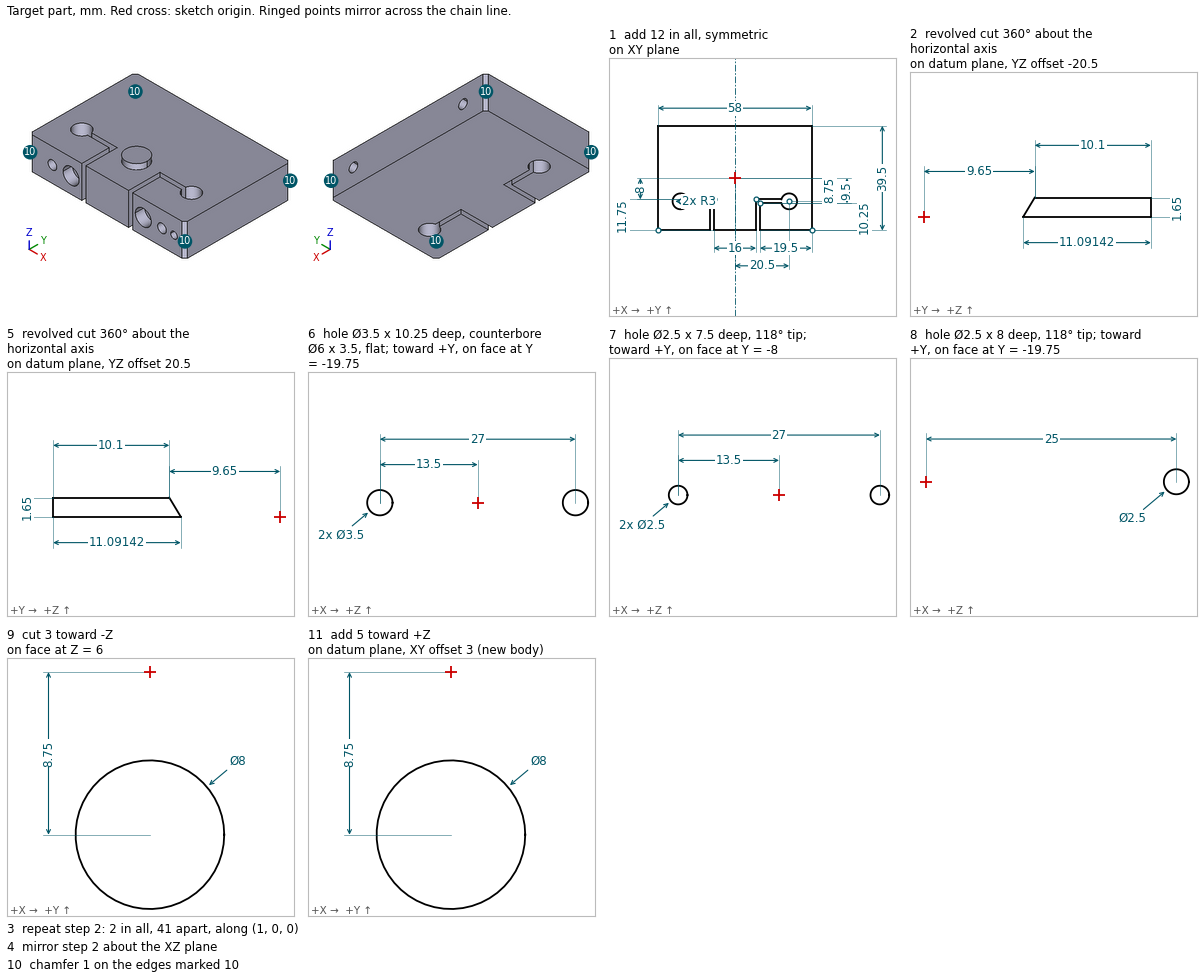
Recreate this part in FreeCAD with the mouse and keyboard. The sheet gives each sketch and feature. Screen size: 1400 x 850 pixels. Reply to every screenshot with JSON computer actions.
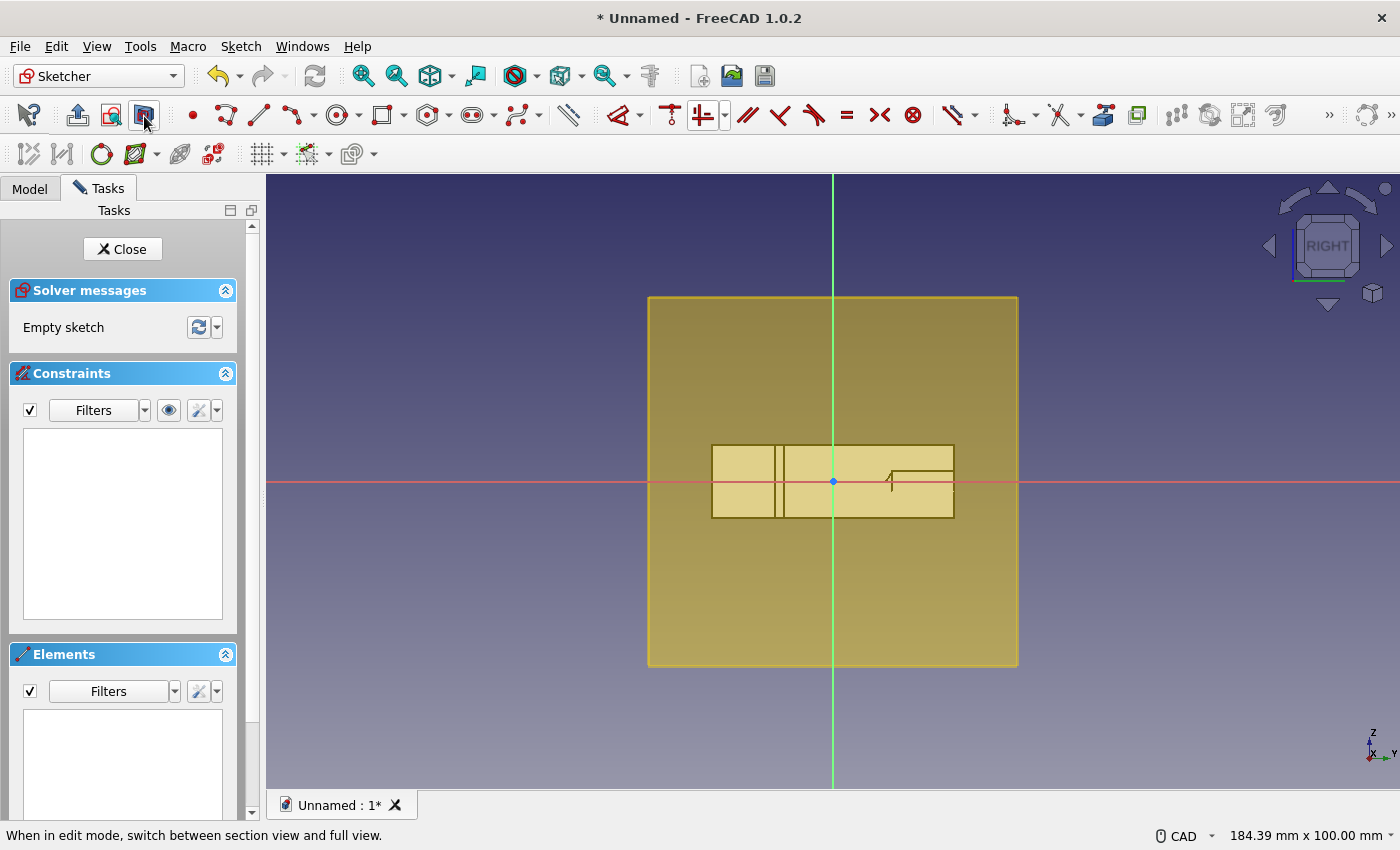
{"action": "scroll", "coordinate": [774, 475], "scroll_direction": "up", "scroll_amount": 8}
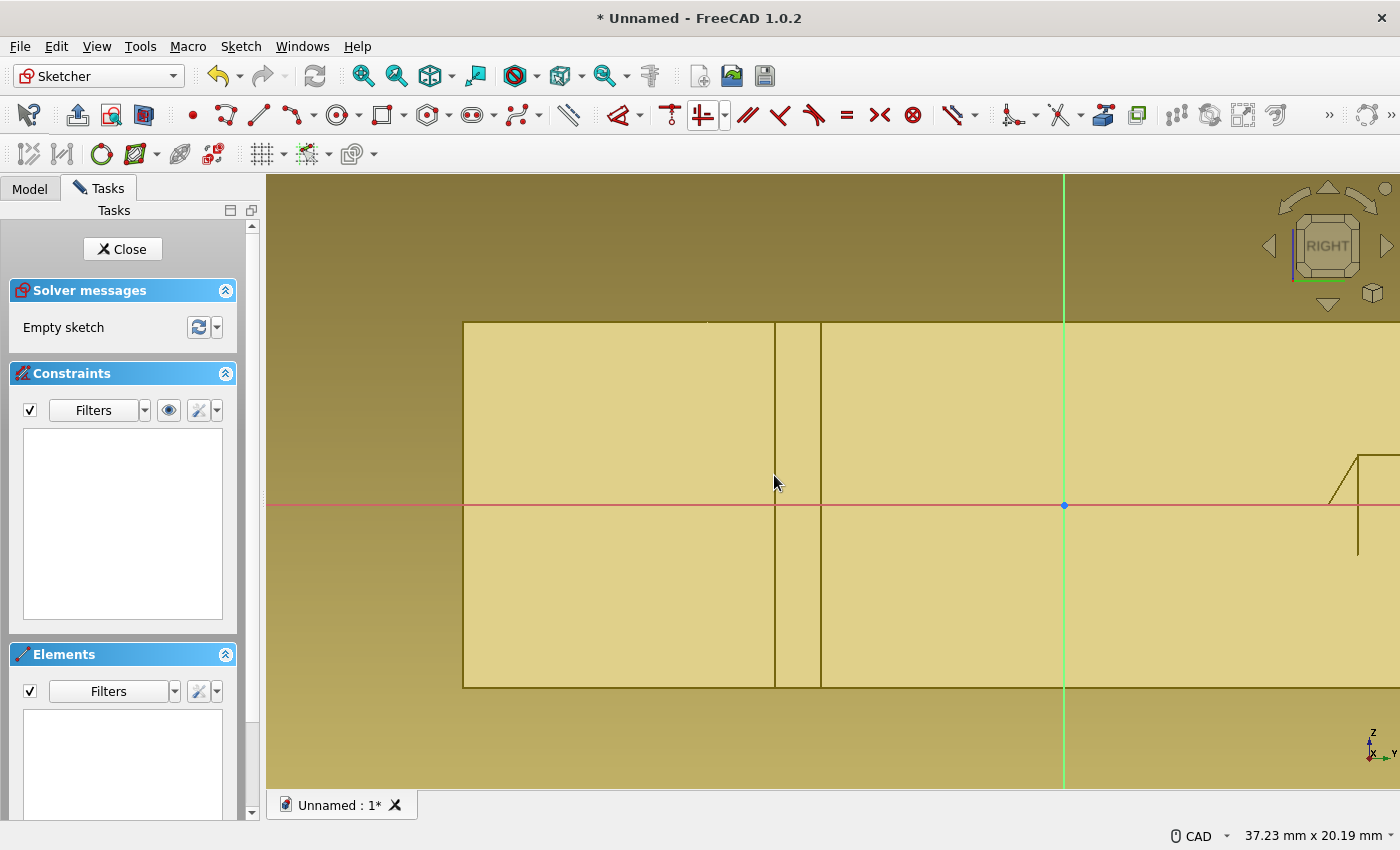
{"action": "left_click", "coordinate": [226, 116]}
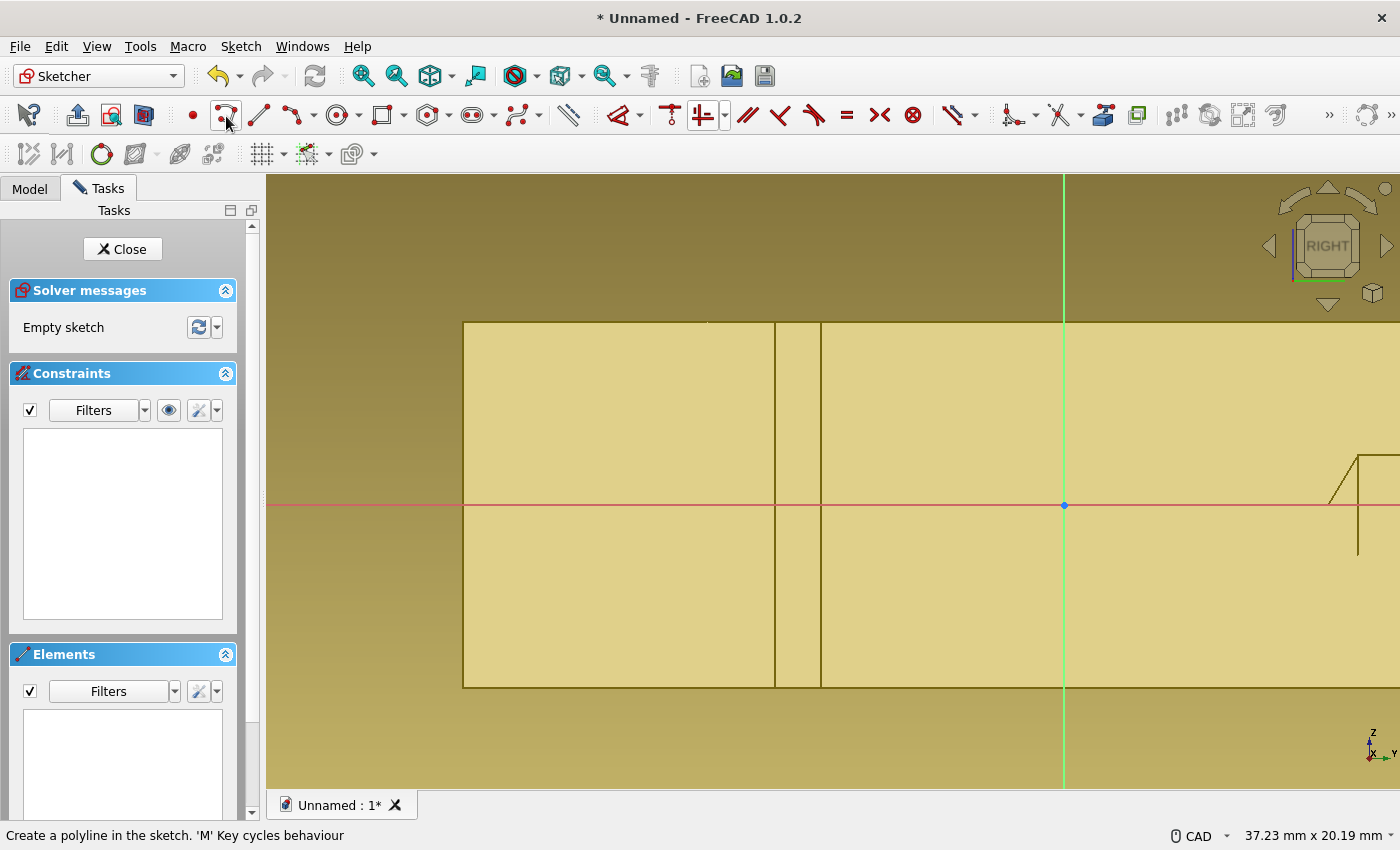
{"action": "left_click", "coordinate": [801, 505]}
{"action": "left_click", "coordinate": [771, 455]}
{"action": "left_click", "coordinate": [463, 455]}
{"action": "left_click", "coordinate": [463, 496]}
{"action": "left_click", "coordinate": [801, 505]}
{"action": "key", "text": "Escape"}
{"action": "key", "text": "Escape"}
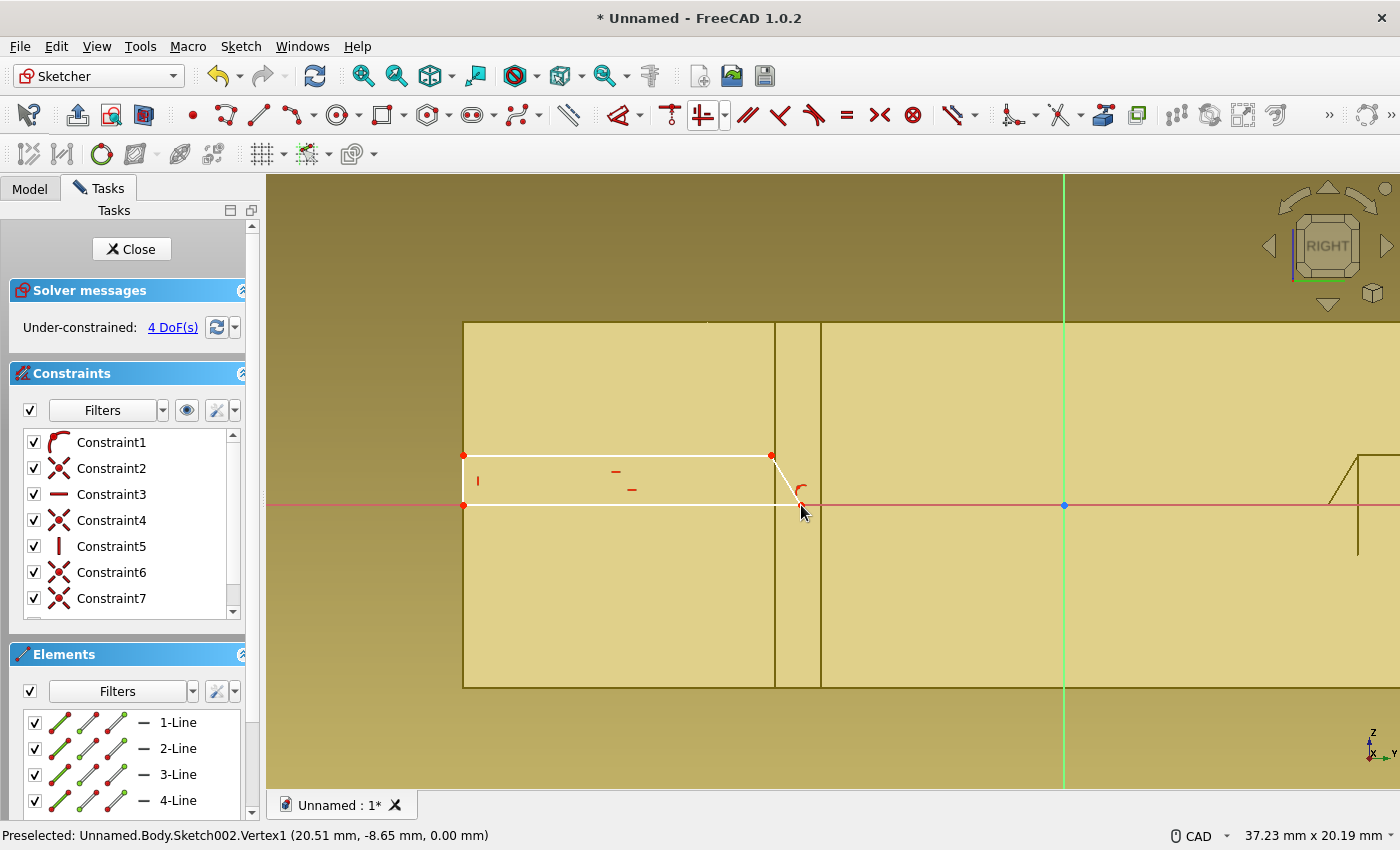
{"action": "left_click", "coordinate": [618, 116]}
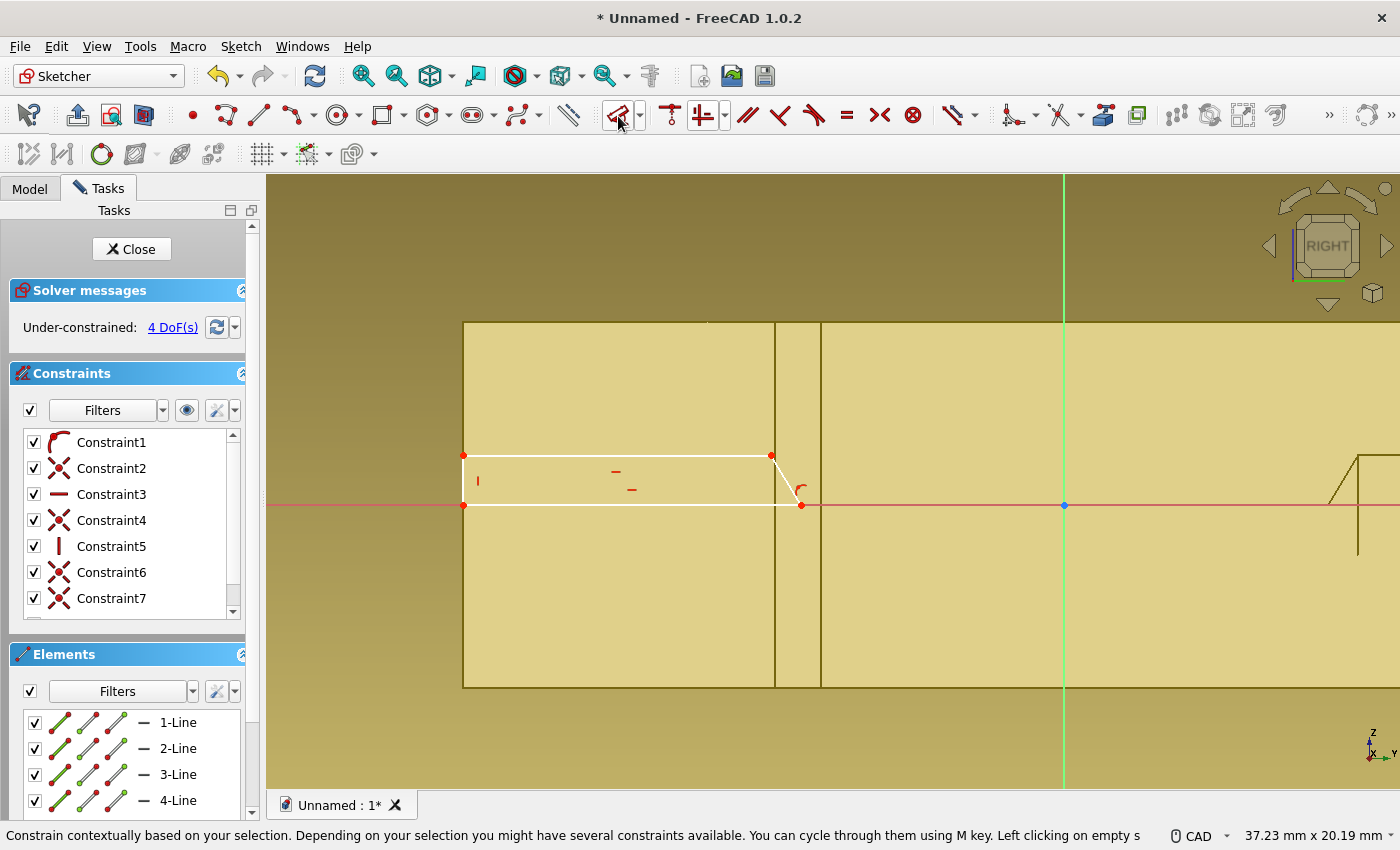
{"action": "left_click", "coordinate": [679, 456]}
{"action": "left_click", "coordinate": [617, 422]}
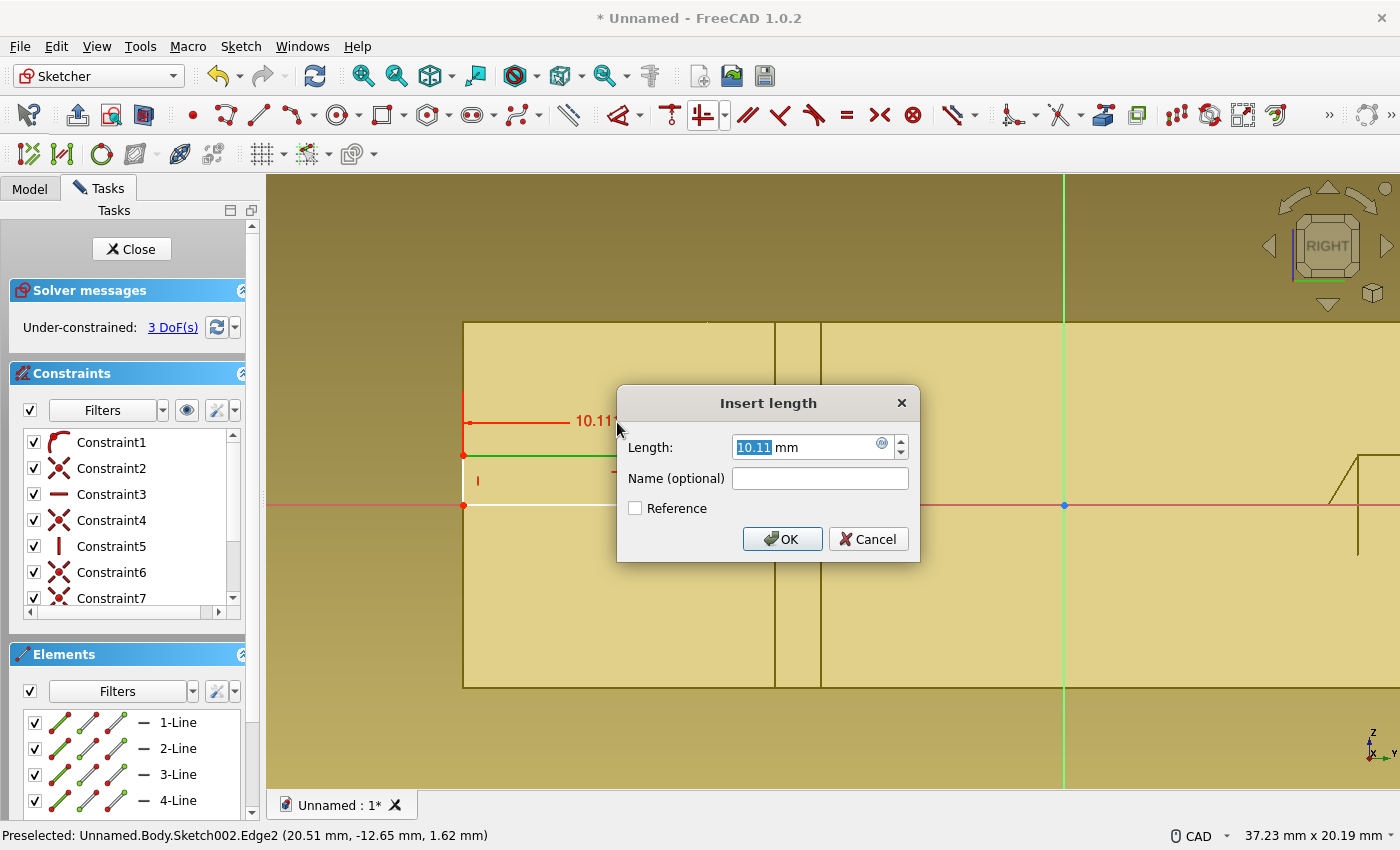
{"action": "type", "text": "10.1"}
{"action": "key", "text": "Return"}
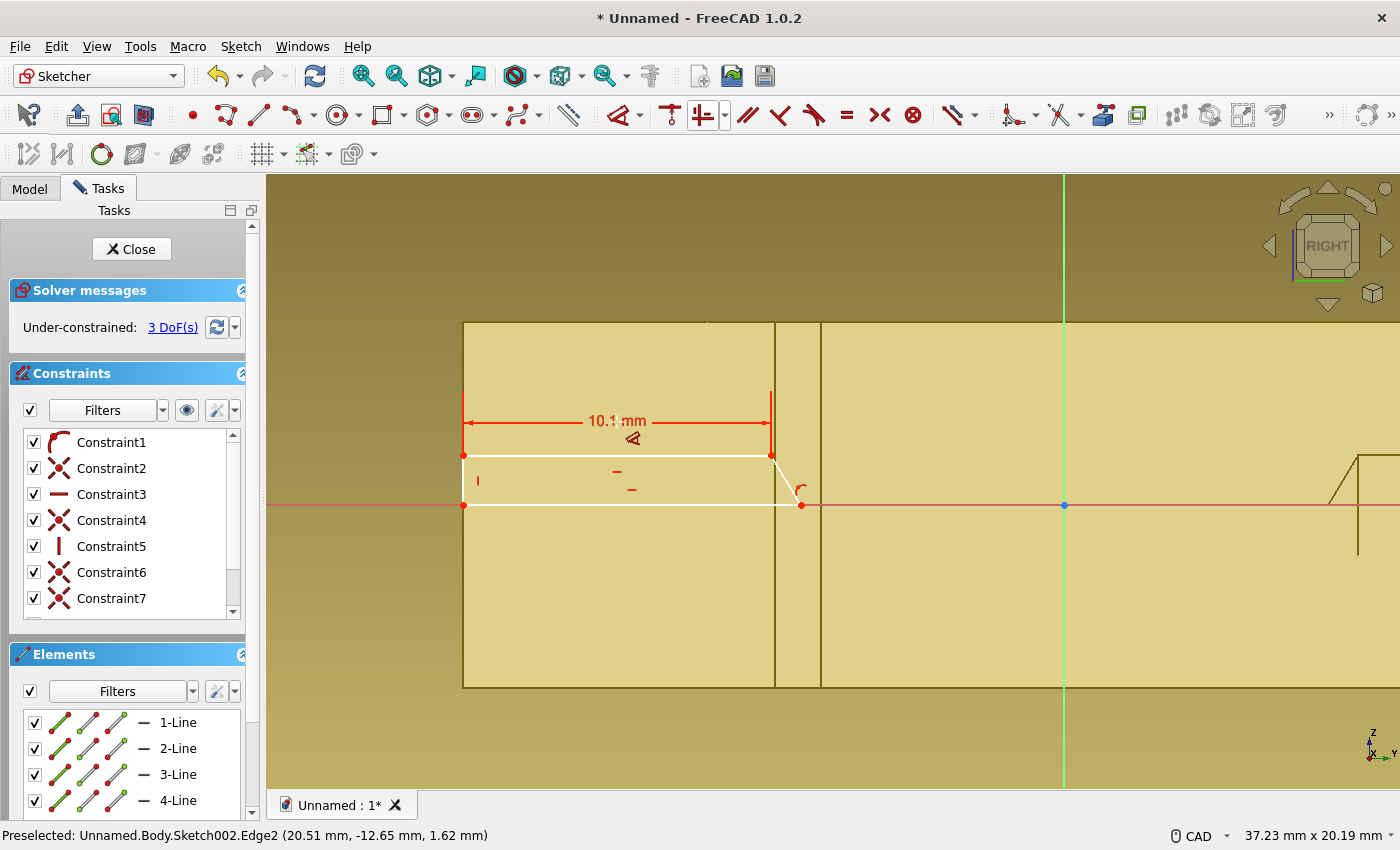
{"action": "left_click", "coordinate": [463, 471]}
{"action": "left_click", "coordinate": [429, 481]}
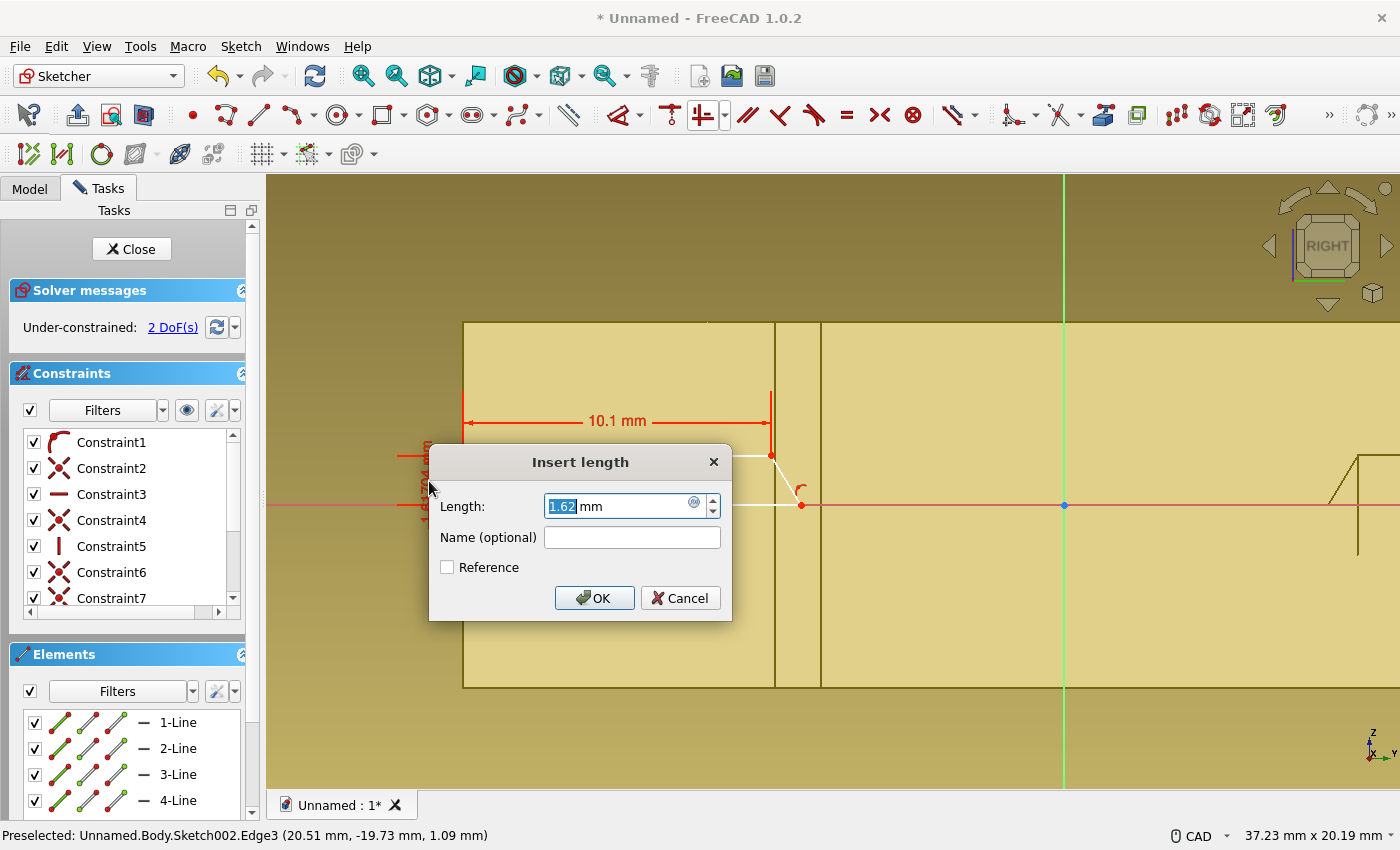
{"action": "type", "text": "1.65"}
{"action": "key", "text": "Return"}